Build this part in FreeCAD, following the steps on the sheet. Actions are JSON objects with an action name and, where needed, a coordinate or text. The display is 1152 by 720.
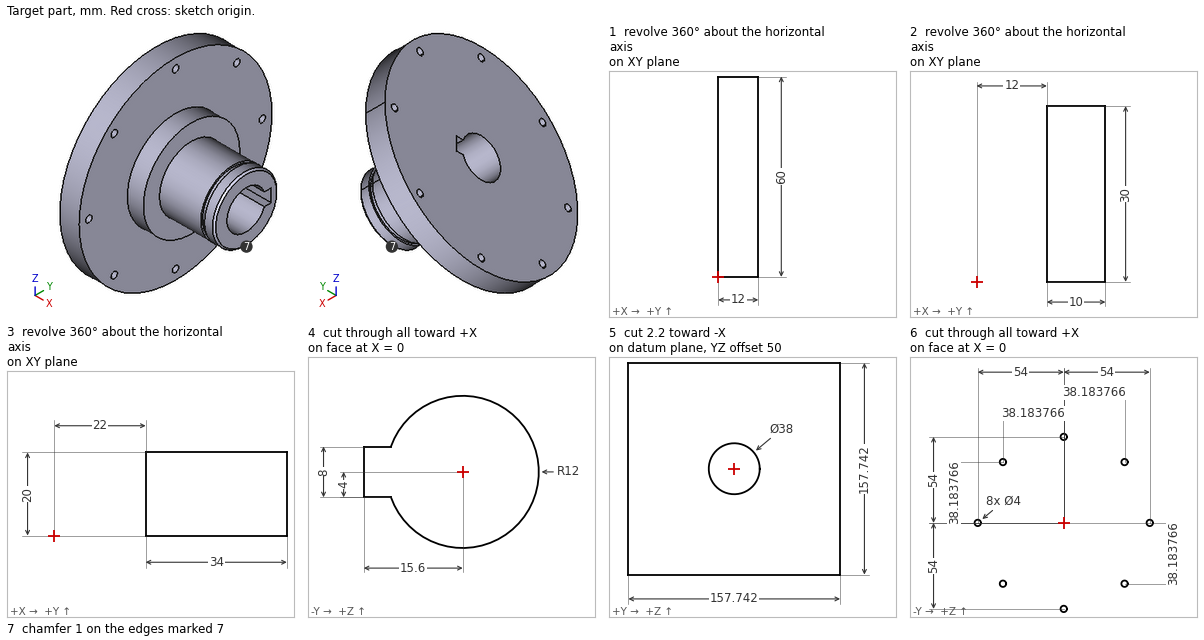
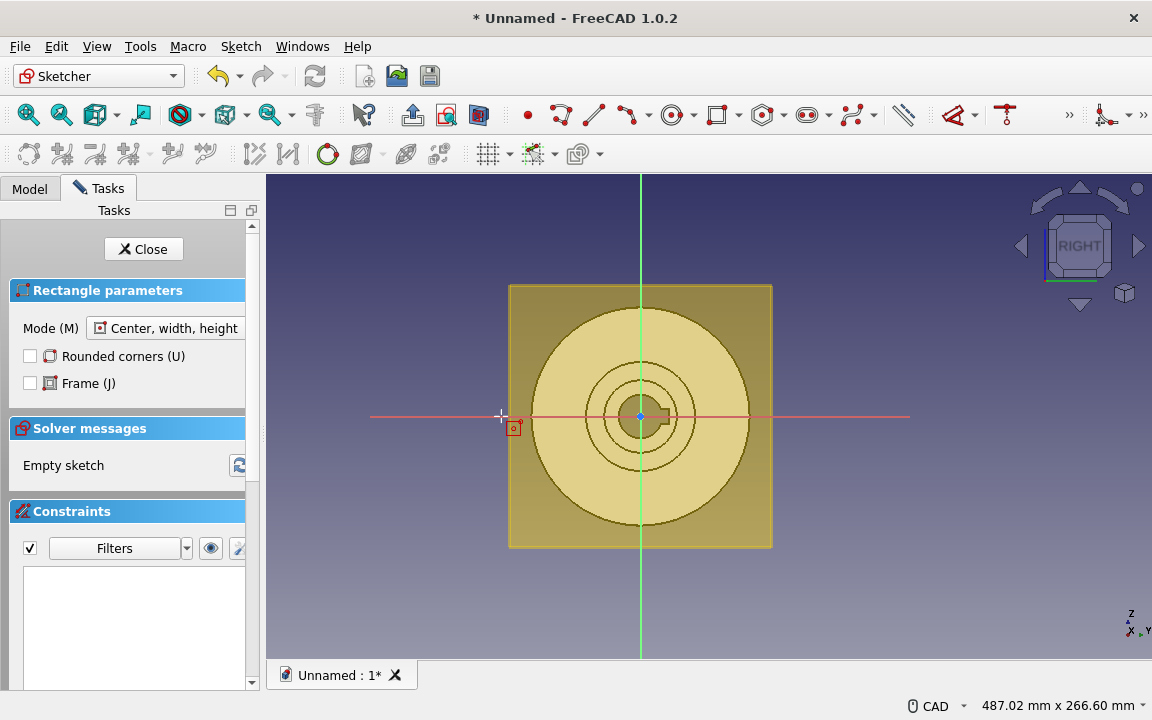
{"action": "left_click", "coordinate": [641, 417]}
{"action": "left_click", "coordinate": [784, 273]}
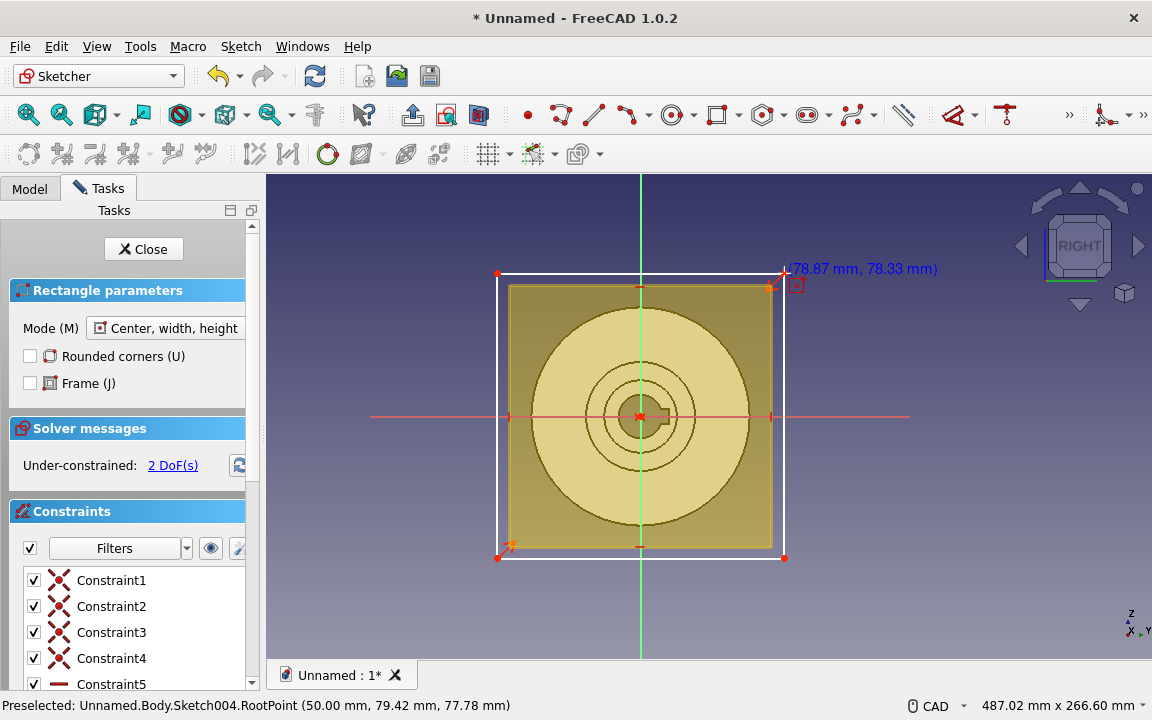
{"action": "left_click", "coordinate": [672, 116]}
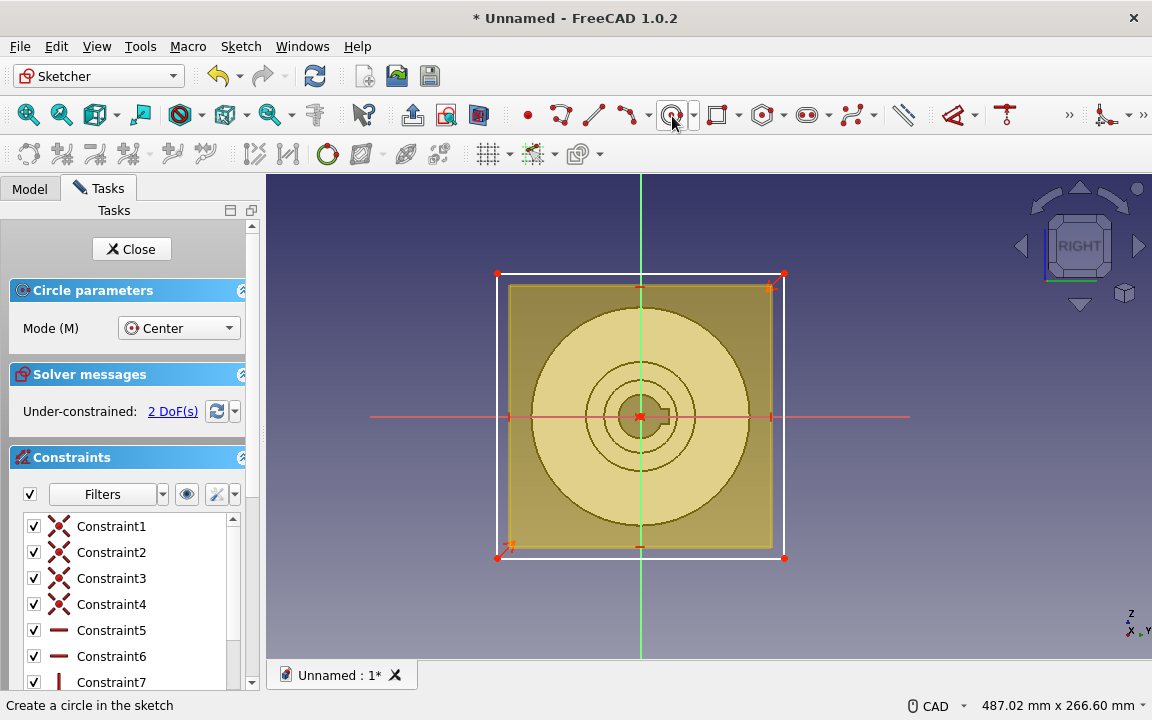
{"action": "left_click", "coordinate": [641, 417]}
{"action": "left_click", "coordinate": [665, 392]}
{"action": "key", "text": "Escape"}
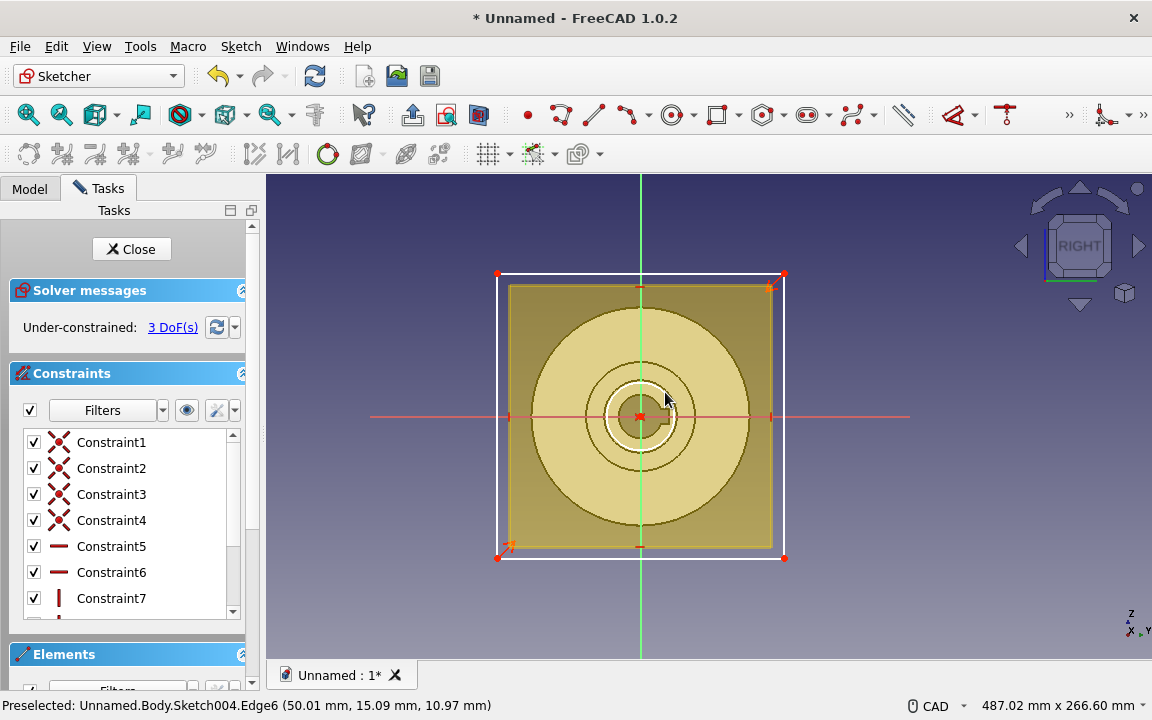
{"action": "left_click", "coordinate": [952, 116]}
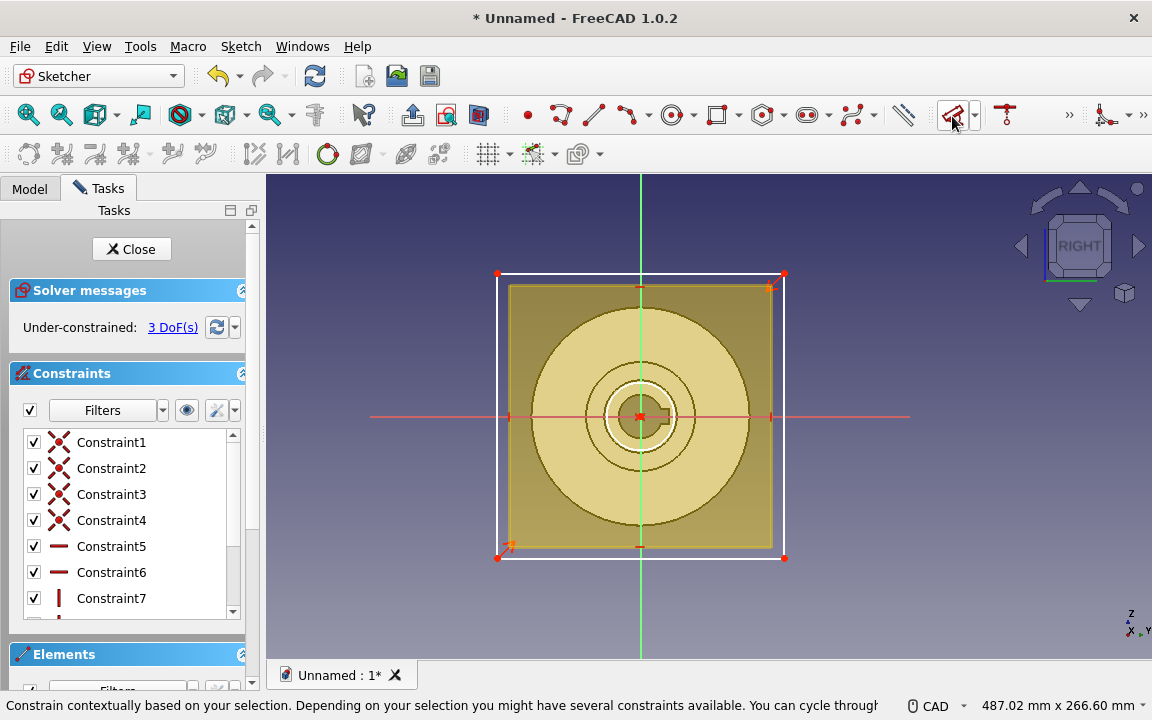
{"action": "left_click", "coordinate": [664, 392]}
{"action": "left_click", "coordinate": [686, 369]}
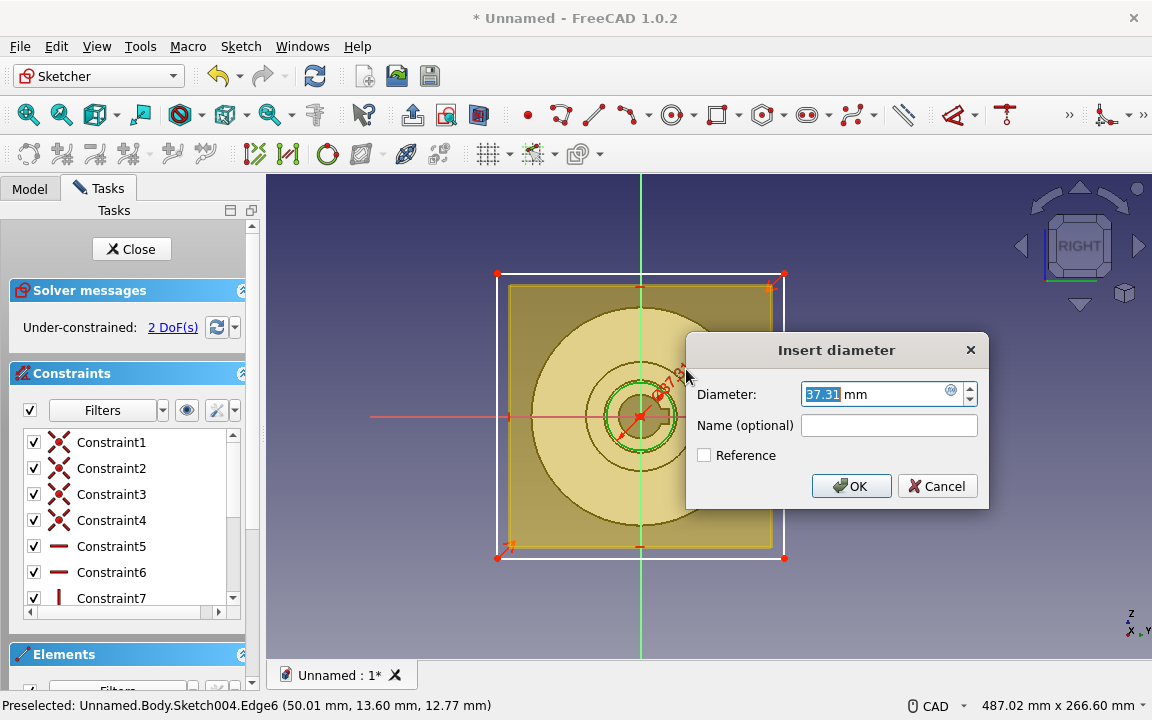
{"action": "type", "text": "38"}
{"action": "key", "text": "Return"}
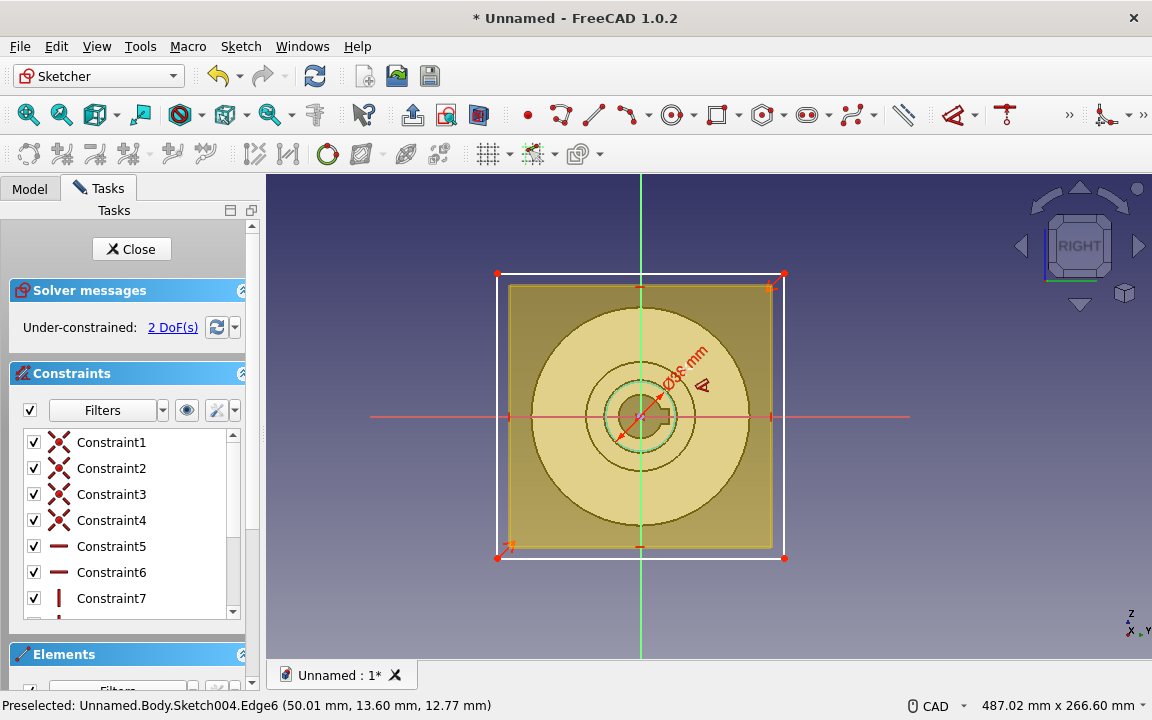
{"action": "left_click", "coordinate": [583, 559]}
{"action": "left_click", "coordinate": [575, 593]}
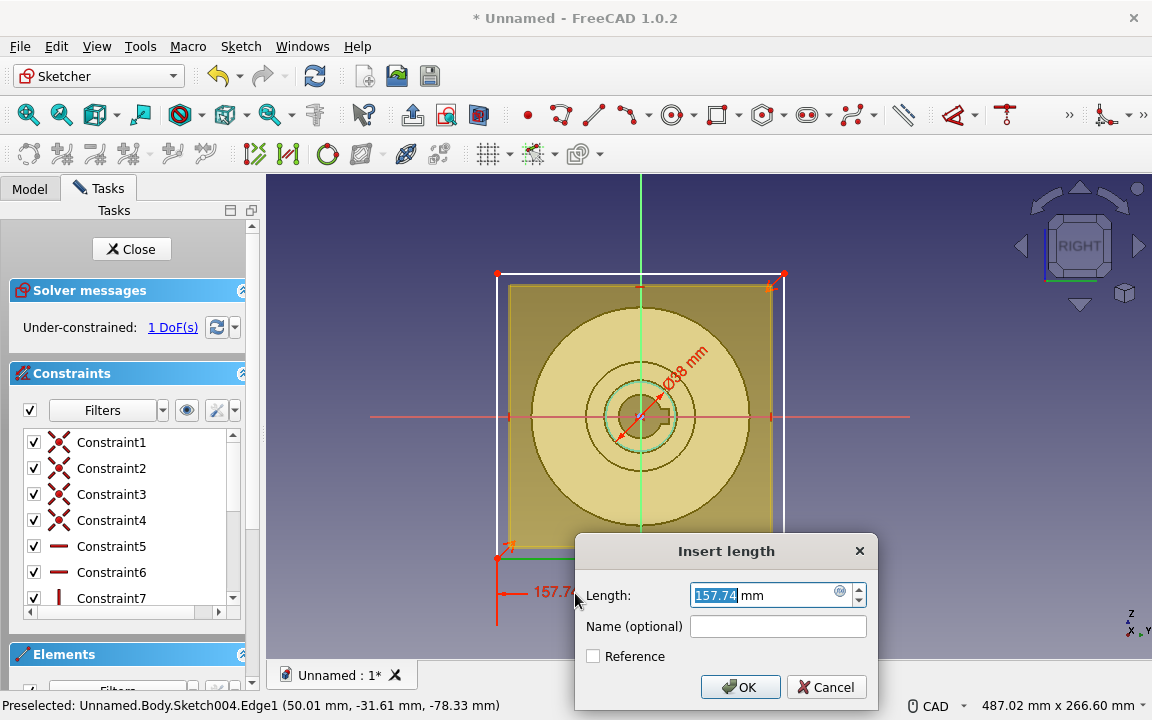
{"action": "type", "text": "157.742"}
{"action": "key", "text": "Return"}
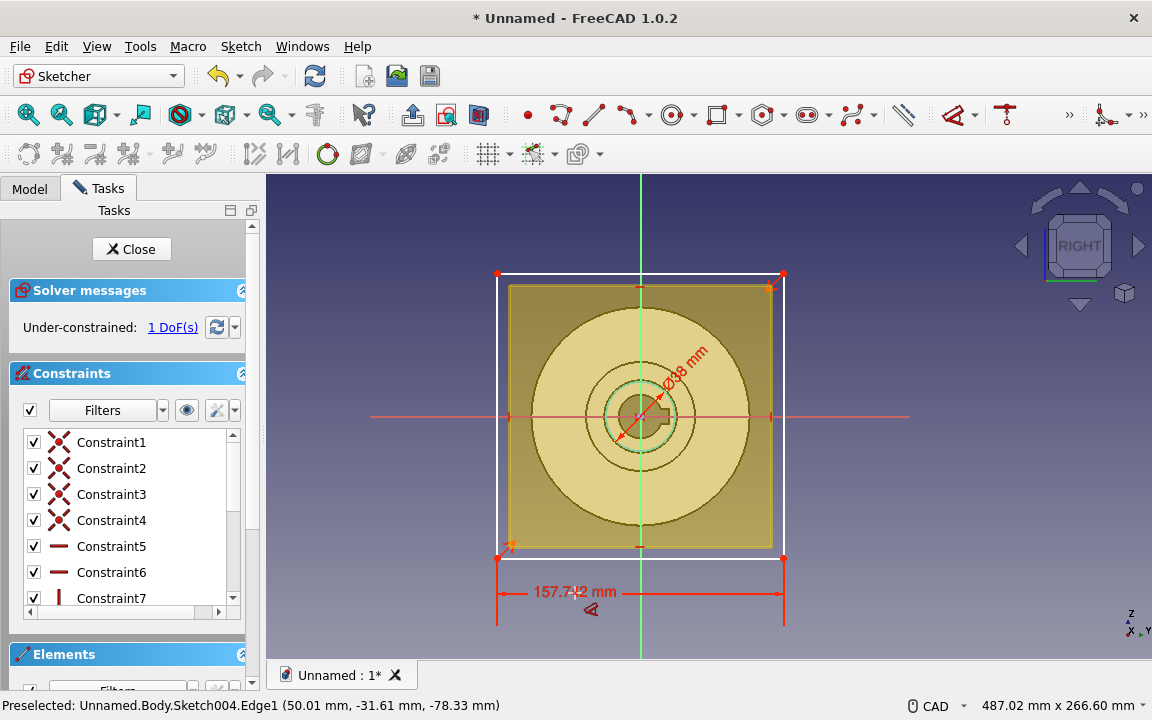
{"action": "left_click", "coordinate": [784, 474]}
{"action": "left_click", "coordinate": [818, 351]}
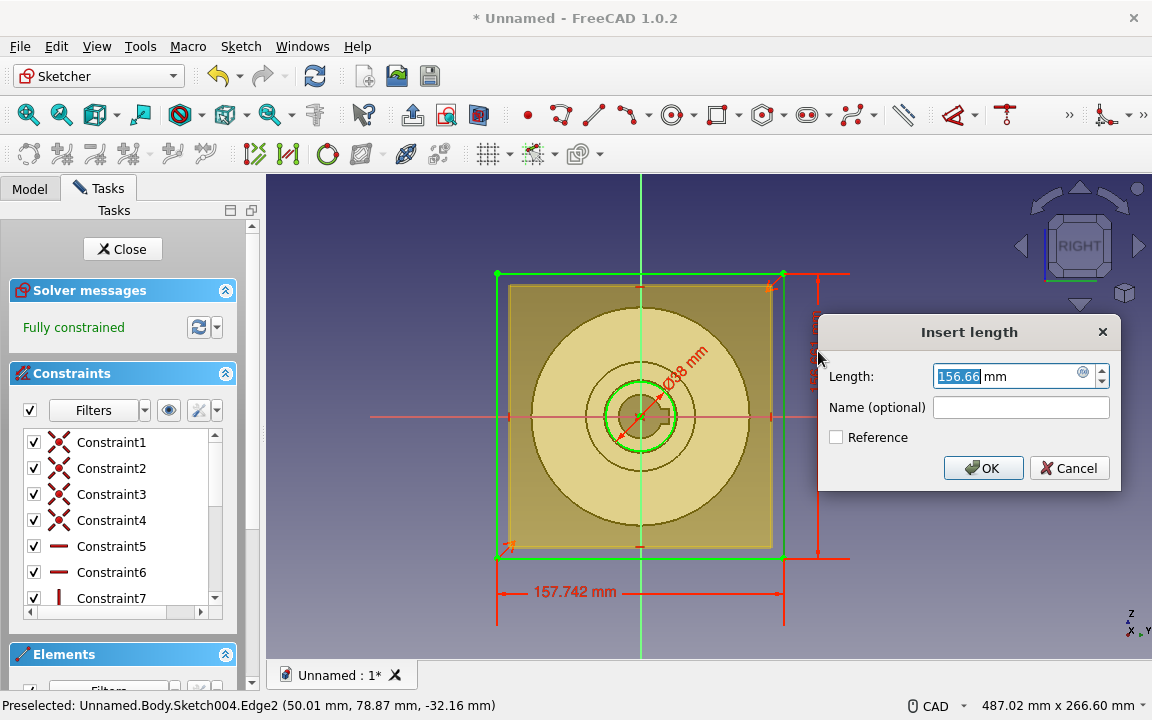
{"action": "type", "text": "157.742"}
{"action": "key", "text": "Return"}
{"action": "key", "text": "Escape"}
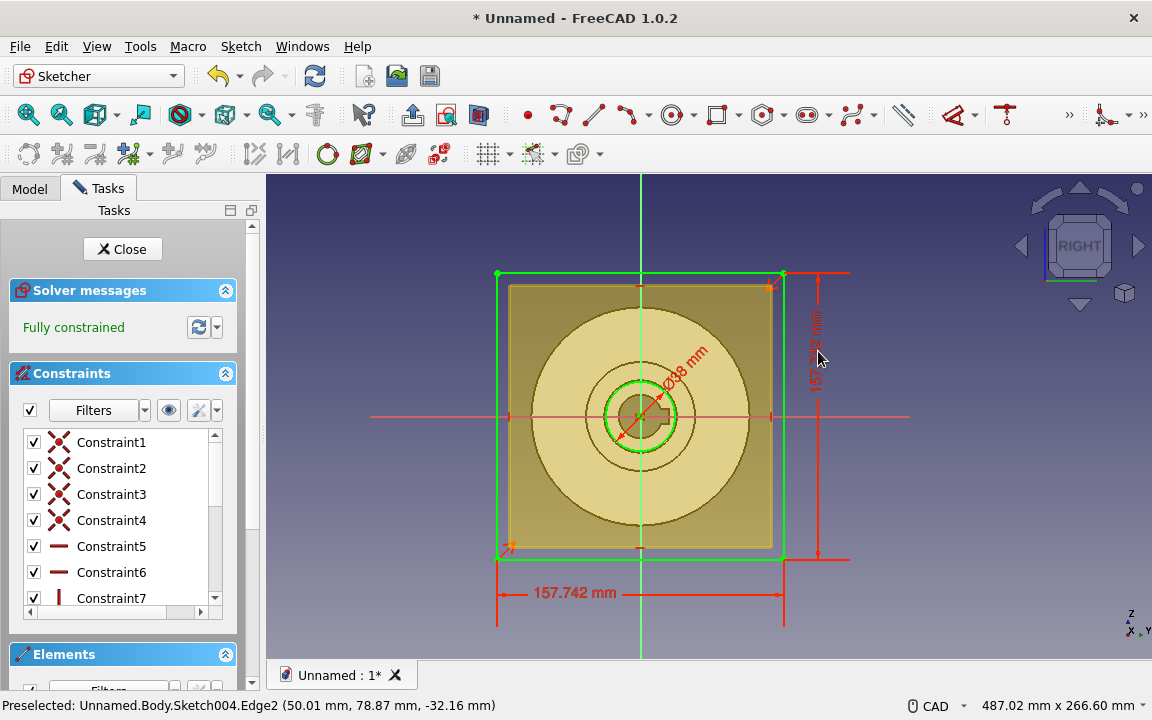
{"action": "left_click", "coordinate": [123, 249]}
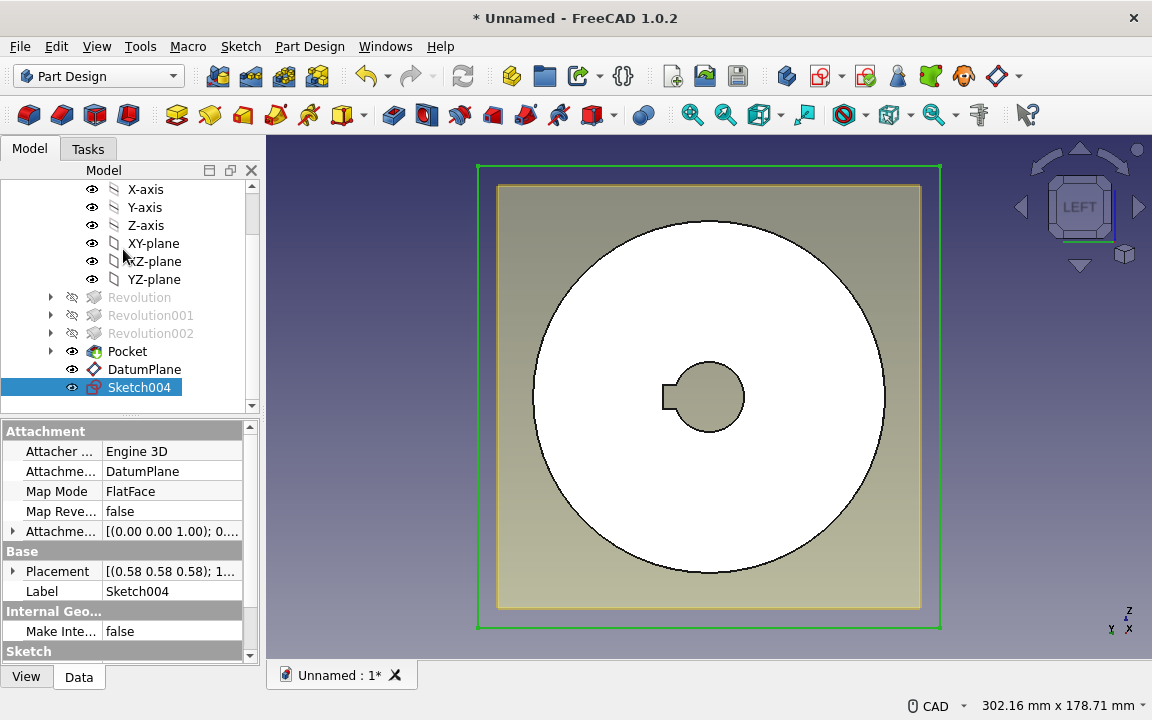
{"action": "left_click", "coordinate": [394, 116]}